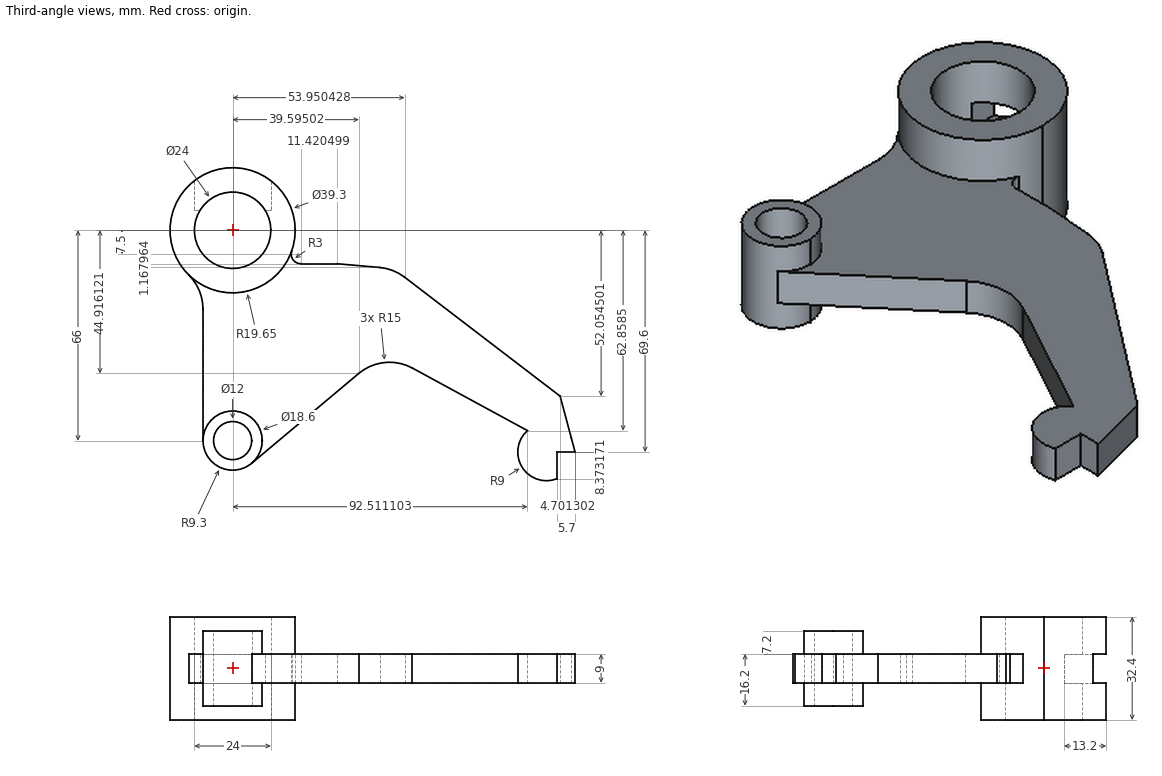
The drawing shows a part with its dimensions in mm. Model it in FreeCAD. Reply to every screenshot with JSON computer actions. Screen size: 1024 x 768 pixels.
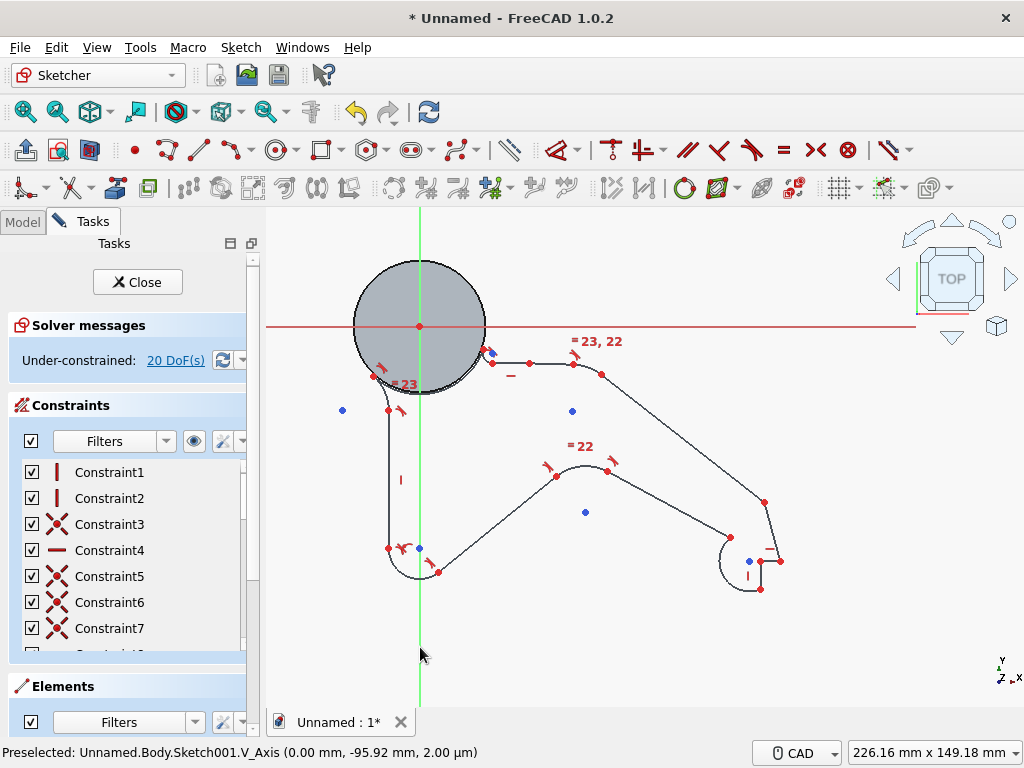
{"action": "key", "text": "d"}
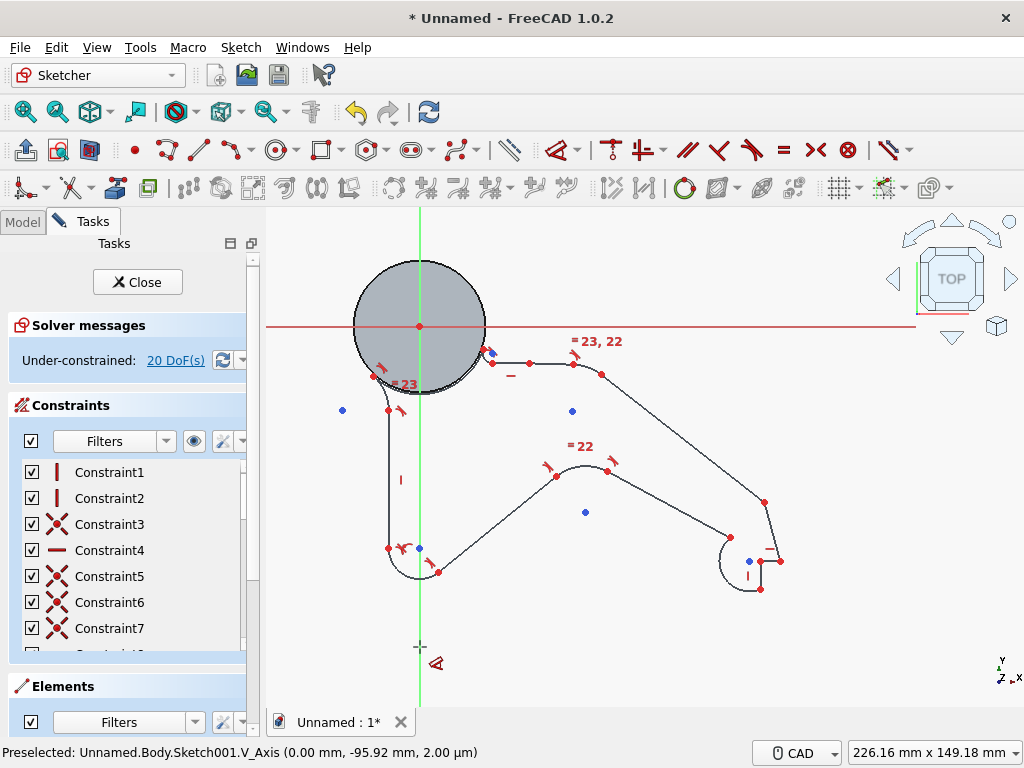
{"action": "scroll", "coordinate": [396, 568], "scroll_direction": "up", "scroll_amount": 2}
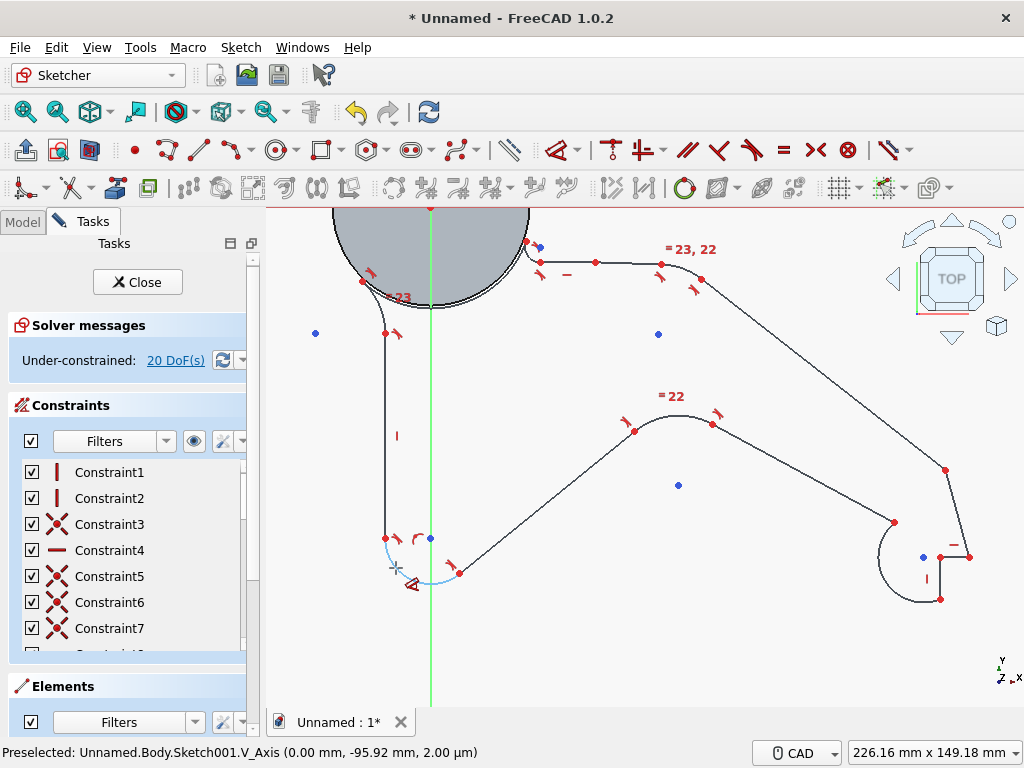
{"action": "left_click", "coordinate": [395, 567]}
{"action": "left_click", "coordinate": [370, 587]}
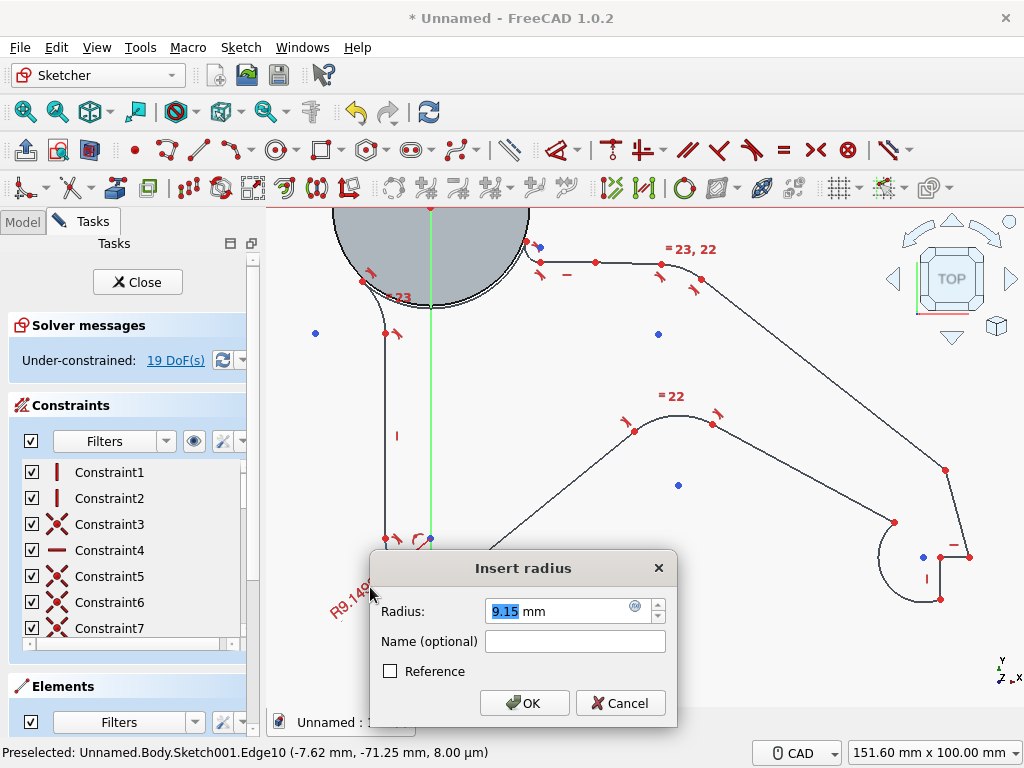
{"action": "type", "text": "9.3"}
{"action": "key", "text": "Return"}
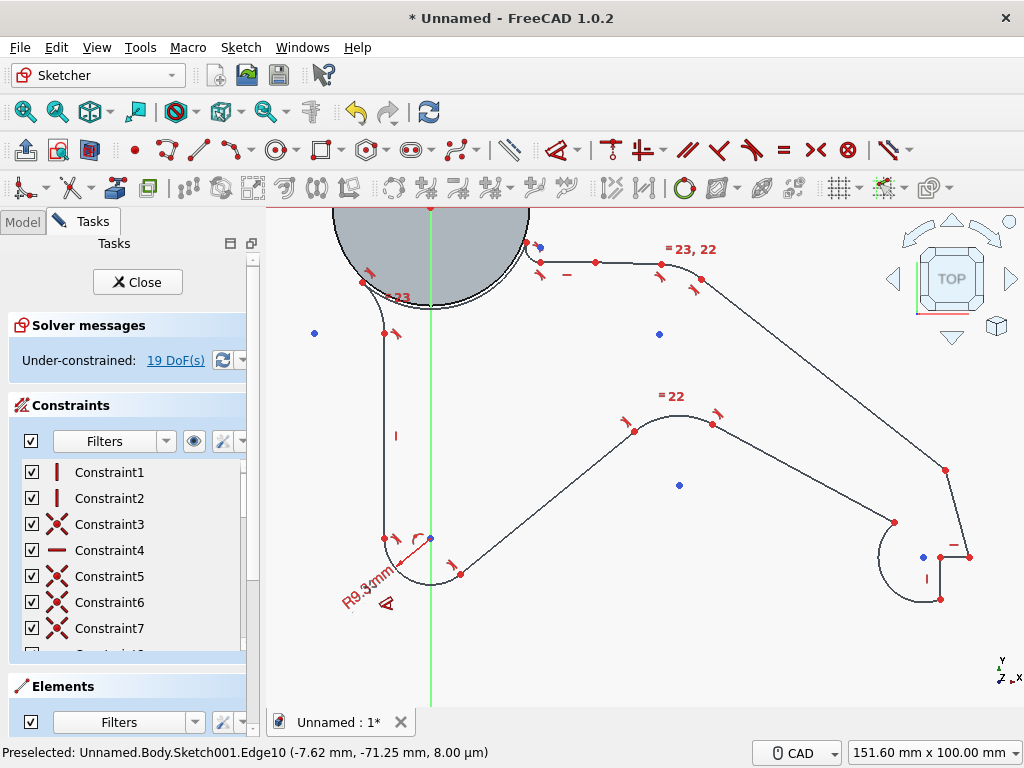
{"action": "left_click", "coordinate": [689, 417]}
{"action": "left_click", "coordinate": [694, 385]}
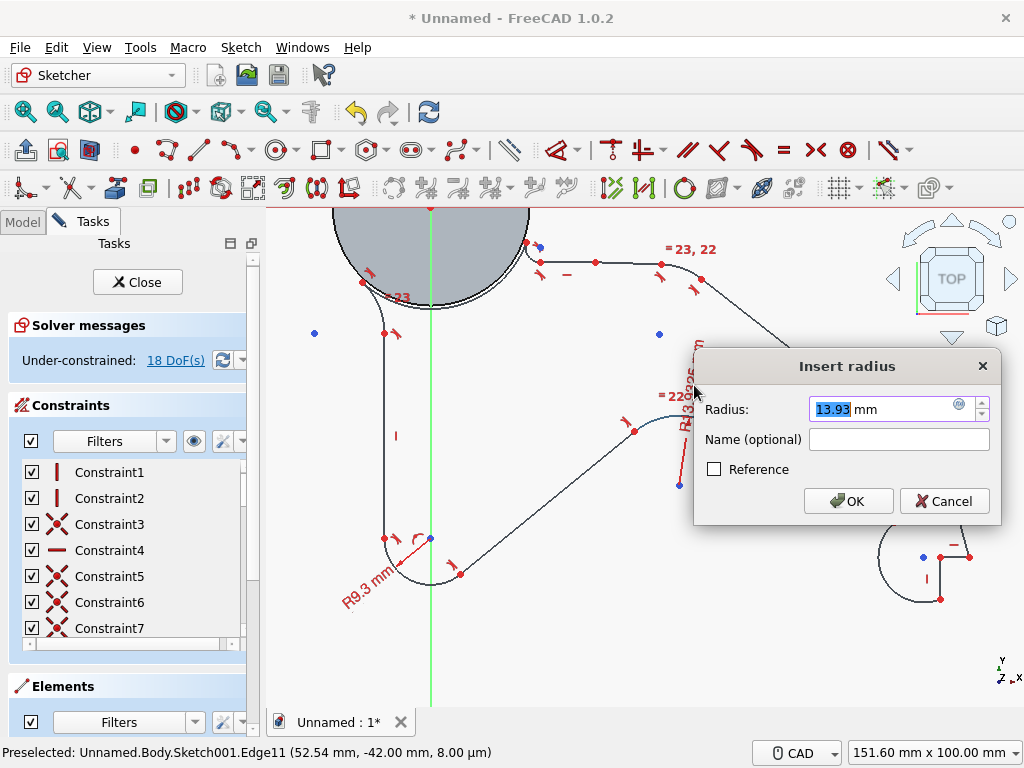
{"action": "type", "text": "15"}
{"action": "key", "text": "Return"}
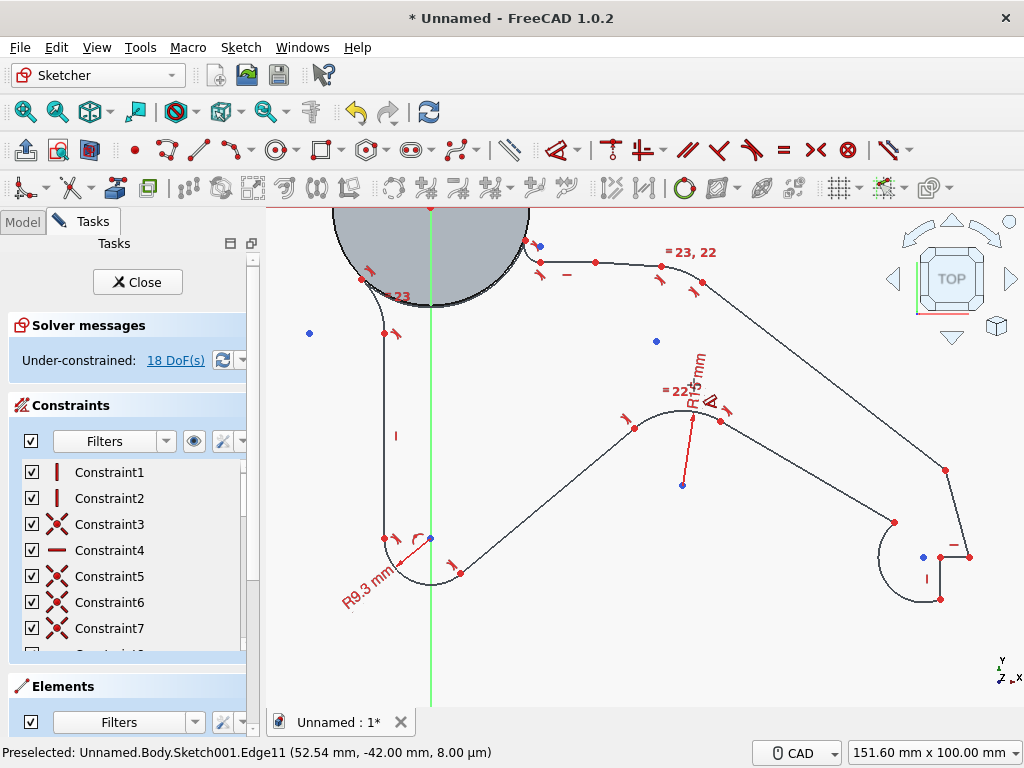
{"action": "scroll", "coordinate": [396, 568], "scroll_direction": "down", "scroll_amount": 2}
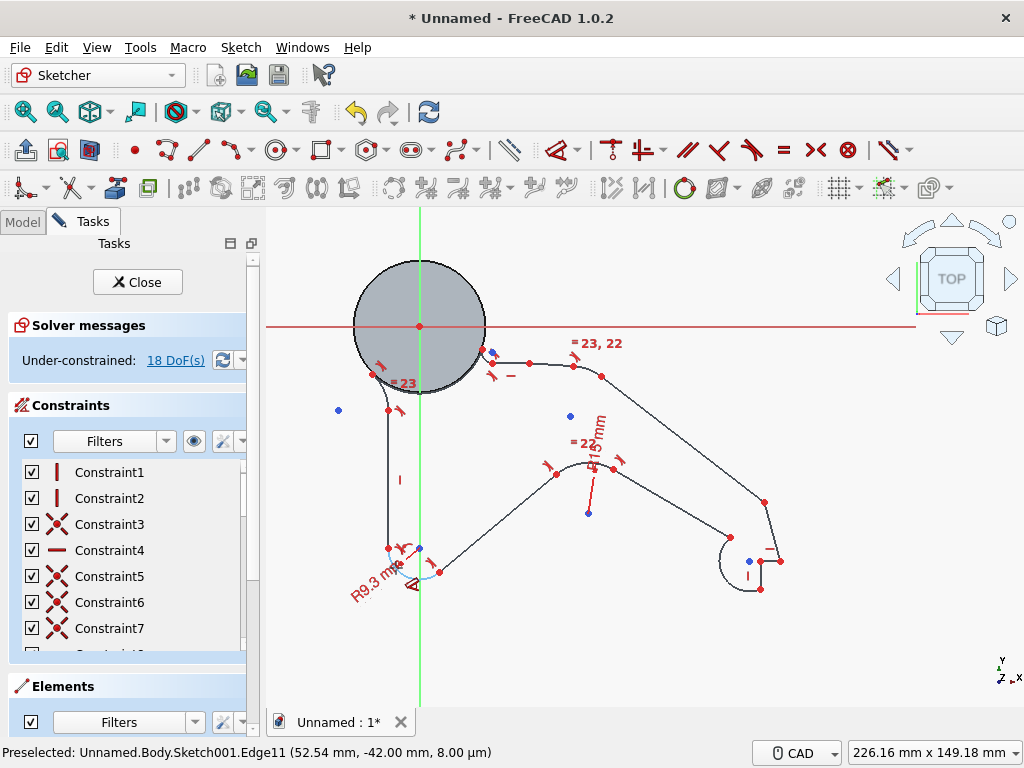
{"action": "scroll", "coordinate": [719, 560], "scroll_direction": "up", "scroll_amount": 2}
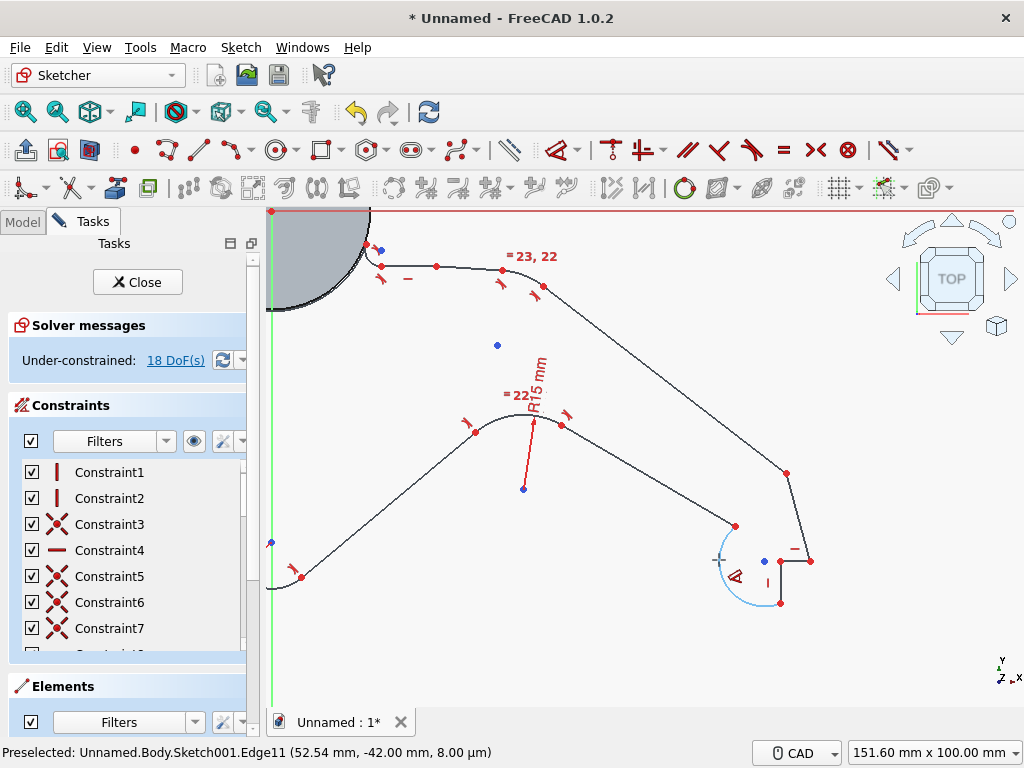
{"action": "left_click", "coordinate": [719, 560]}
{"action": "left_click", "coordinate": [687, 559]}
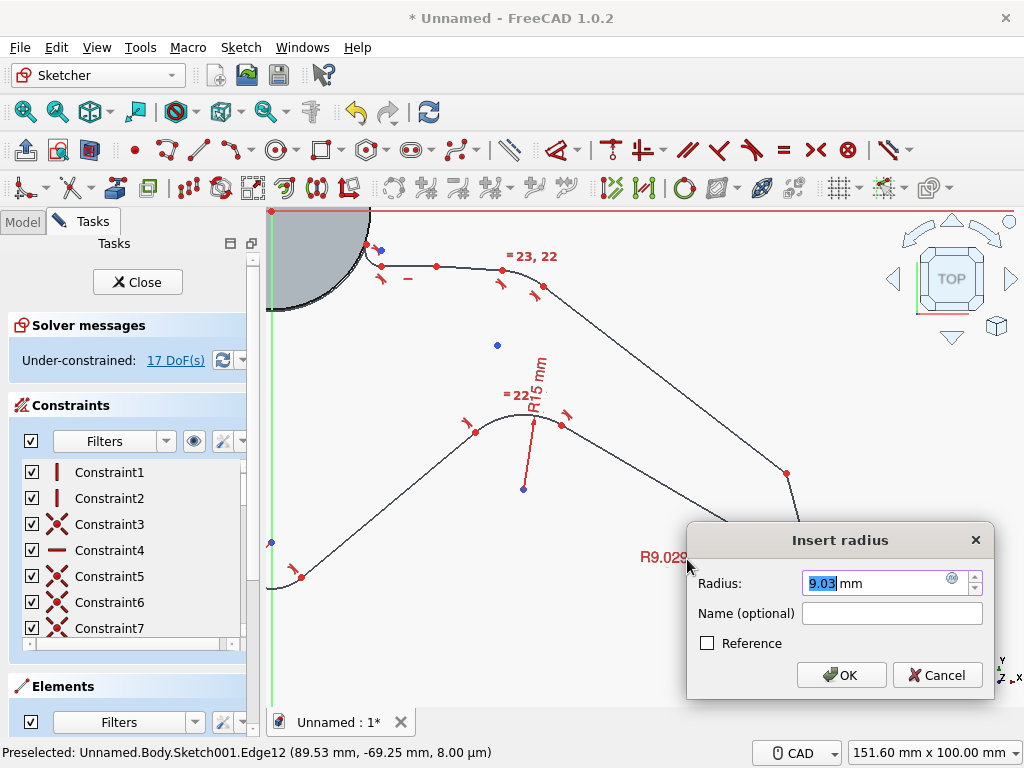
{"action": "type", "text": "9"}
{"action": "key", "text": "Return"}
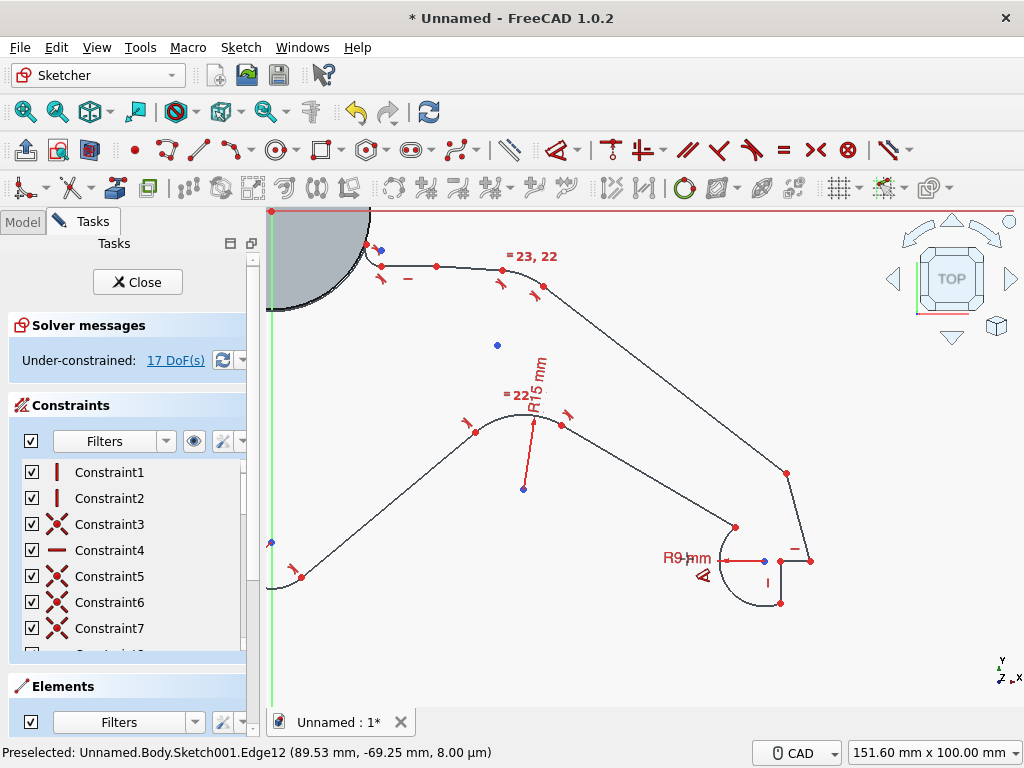
{"action": "scroll", "coordinate": [373, 264], "scroll_direction": "up", "scroll_amount": 5}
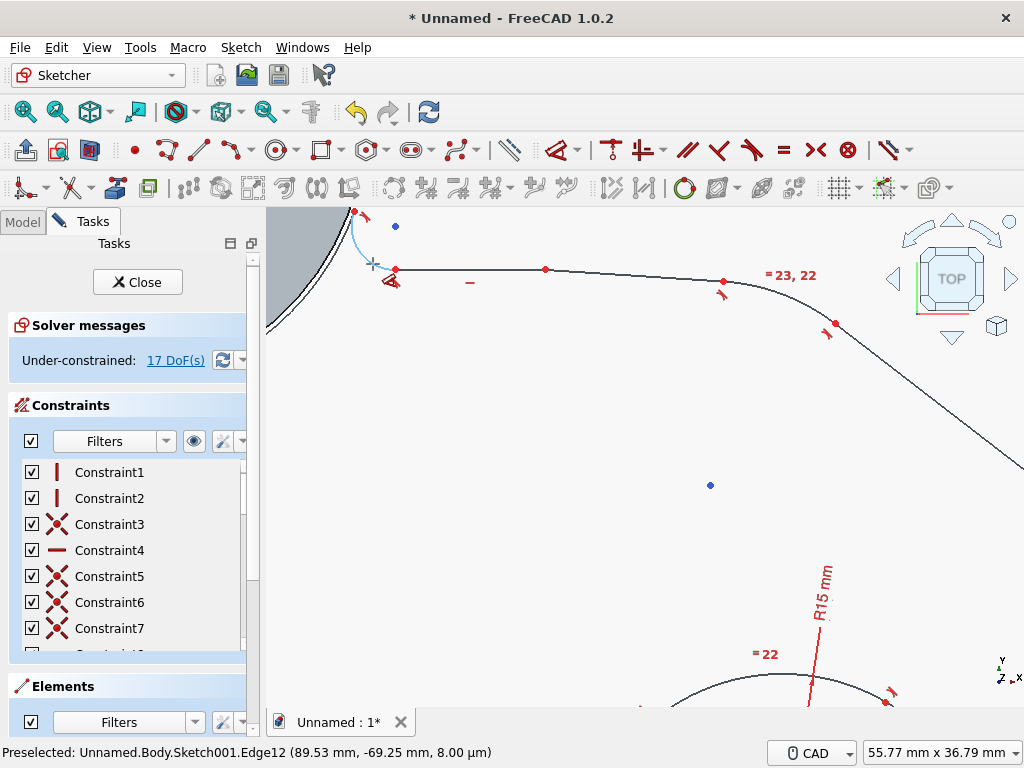
{"action": "left_click", "coordinate": [371, 263]}
{"action": "left_click", "coordinate": [353, 290]}